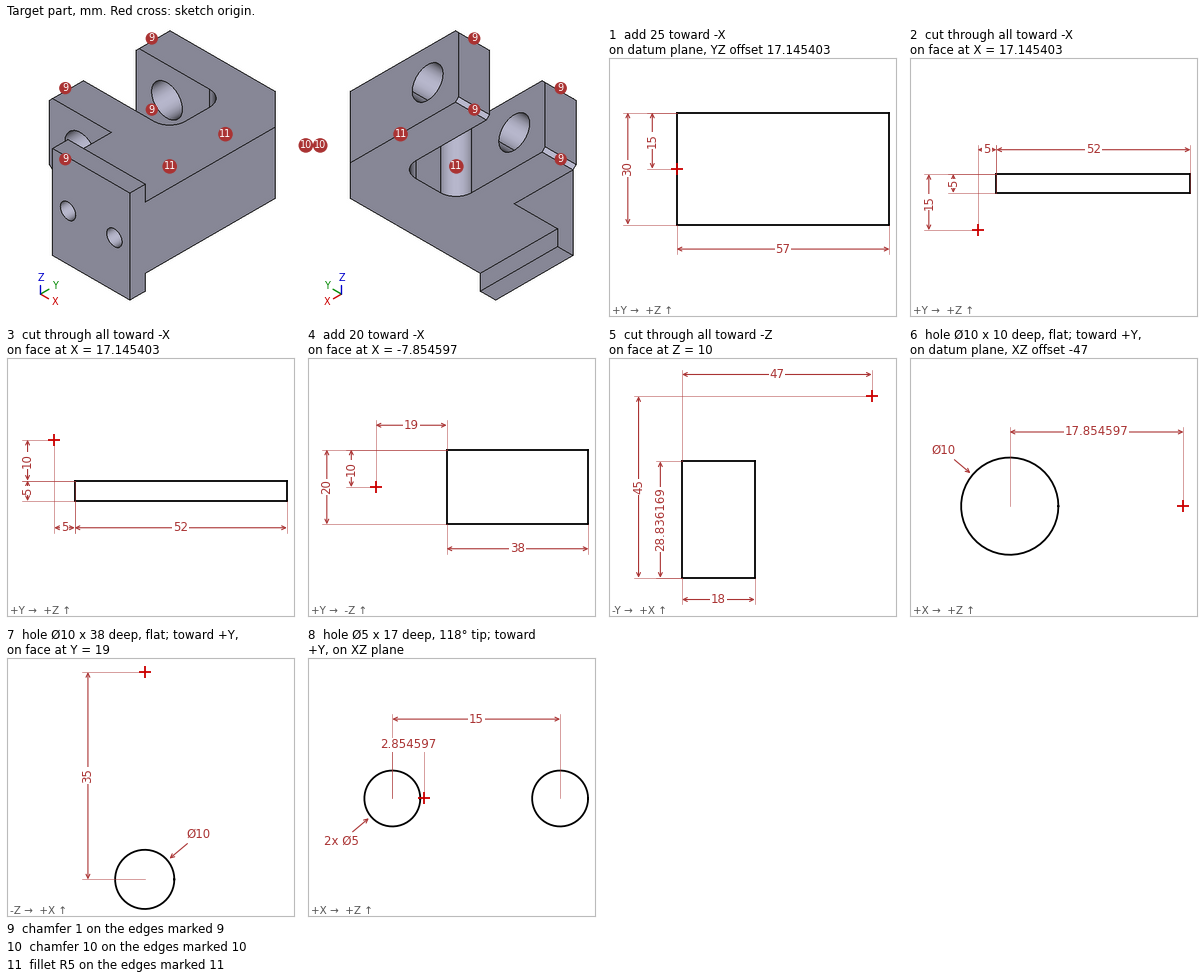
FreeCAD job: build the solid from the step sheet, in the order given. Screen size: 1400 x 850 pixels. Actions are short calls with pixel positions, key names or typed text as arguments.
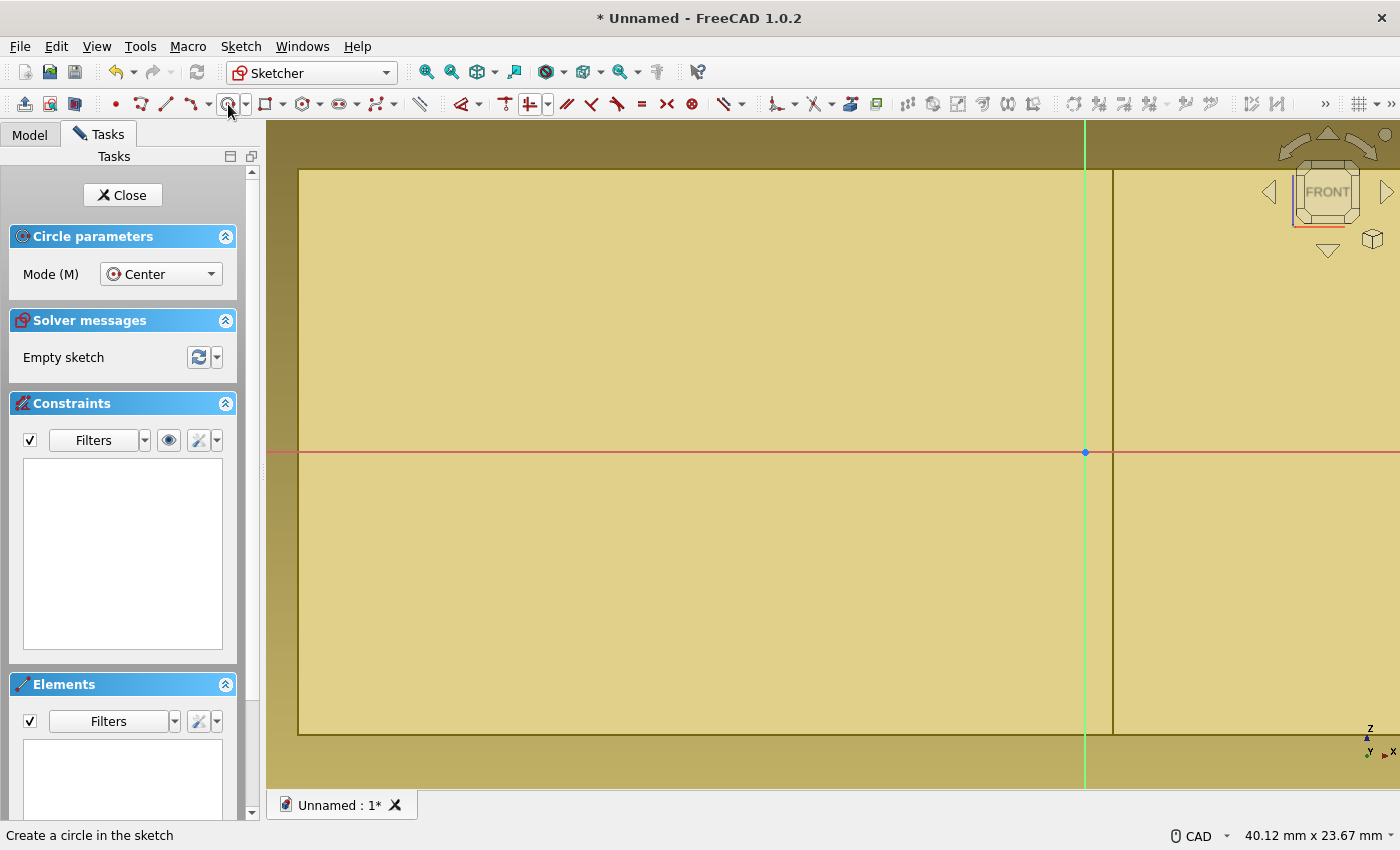
click(581, 452)
click(681, 352)
key(Escape)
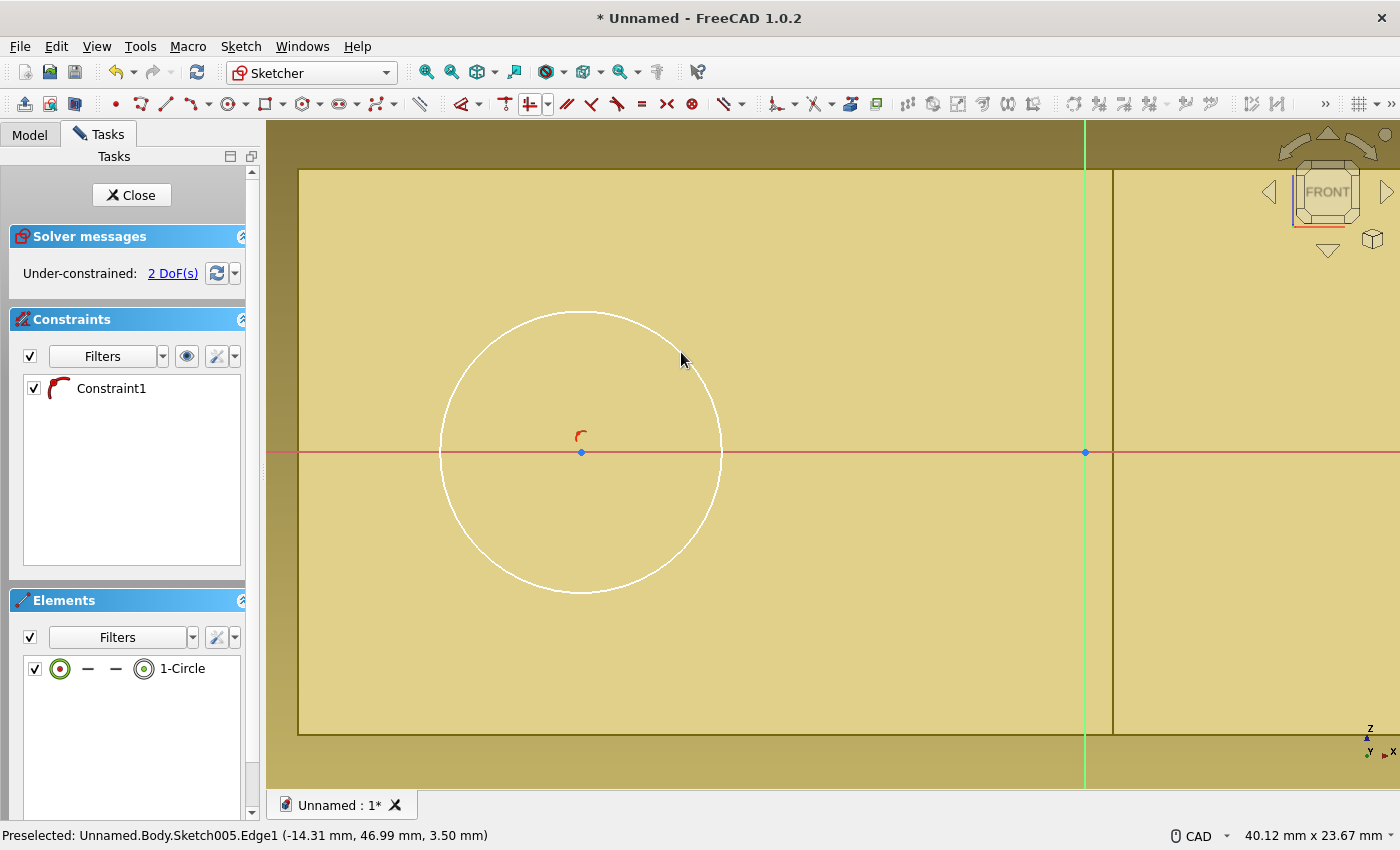
key(d)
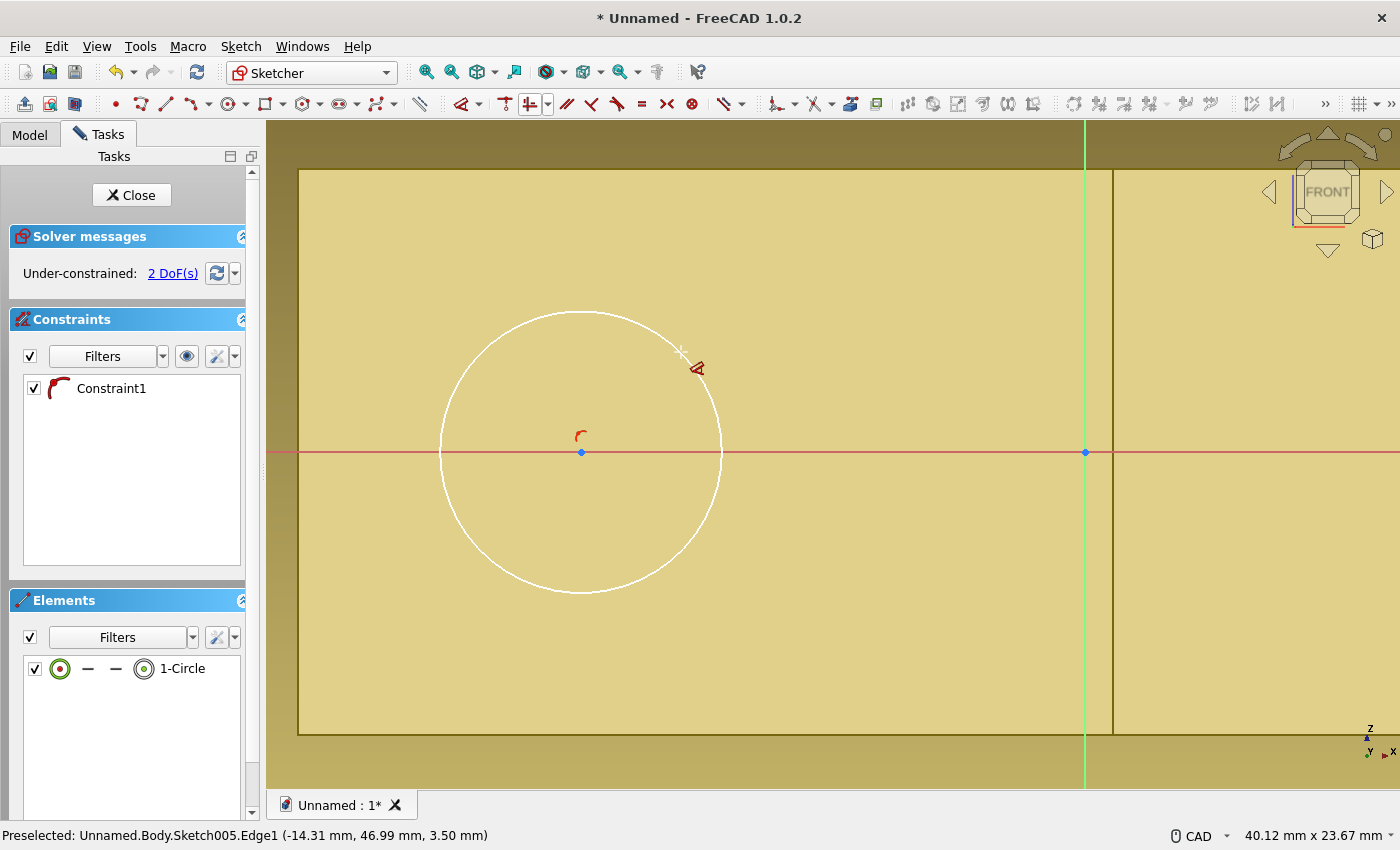
click(680, 352)
click(702, 329)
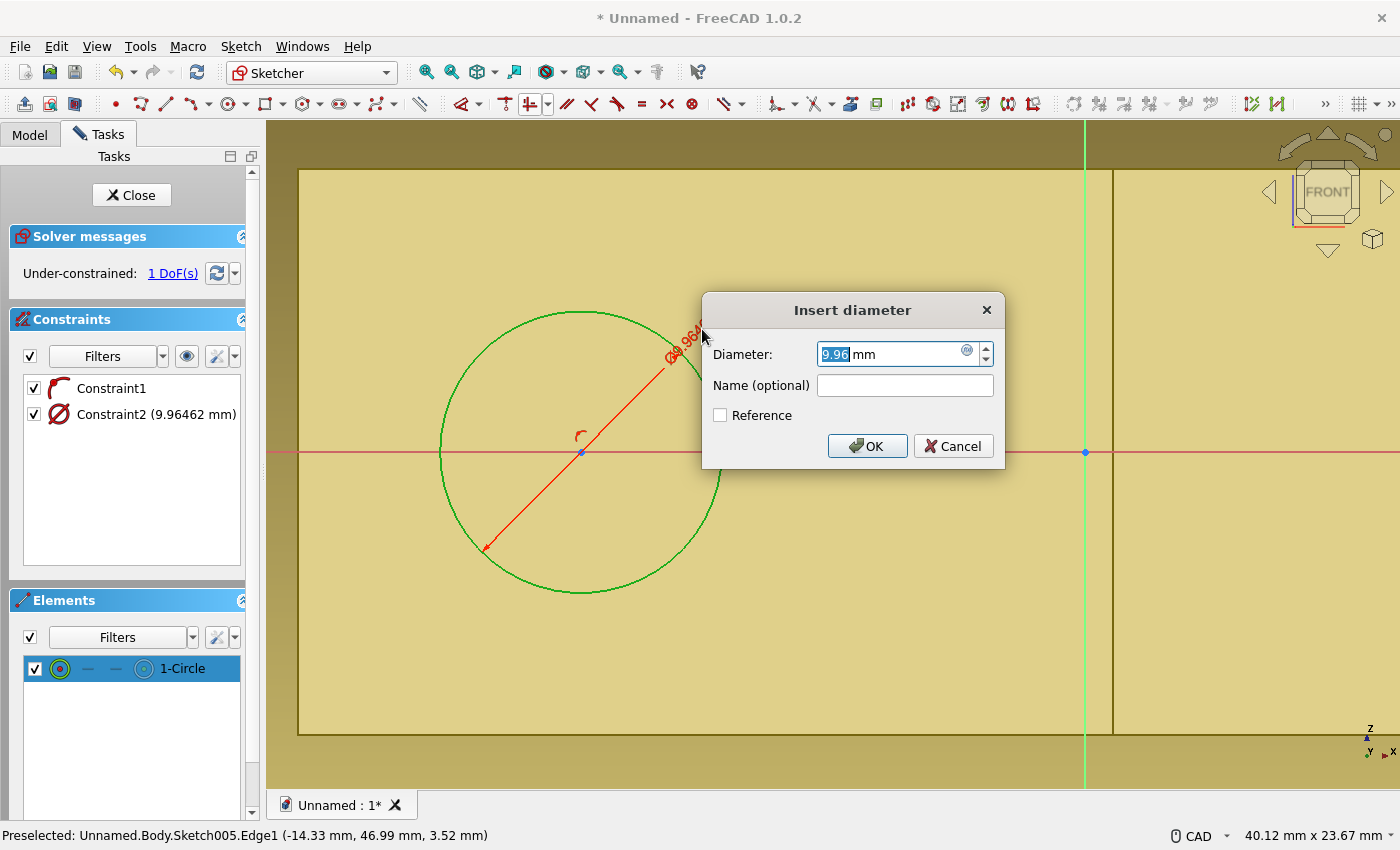
text(10)
key(Return)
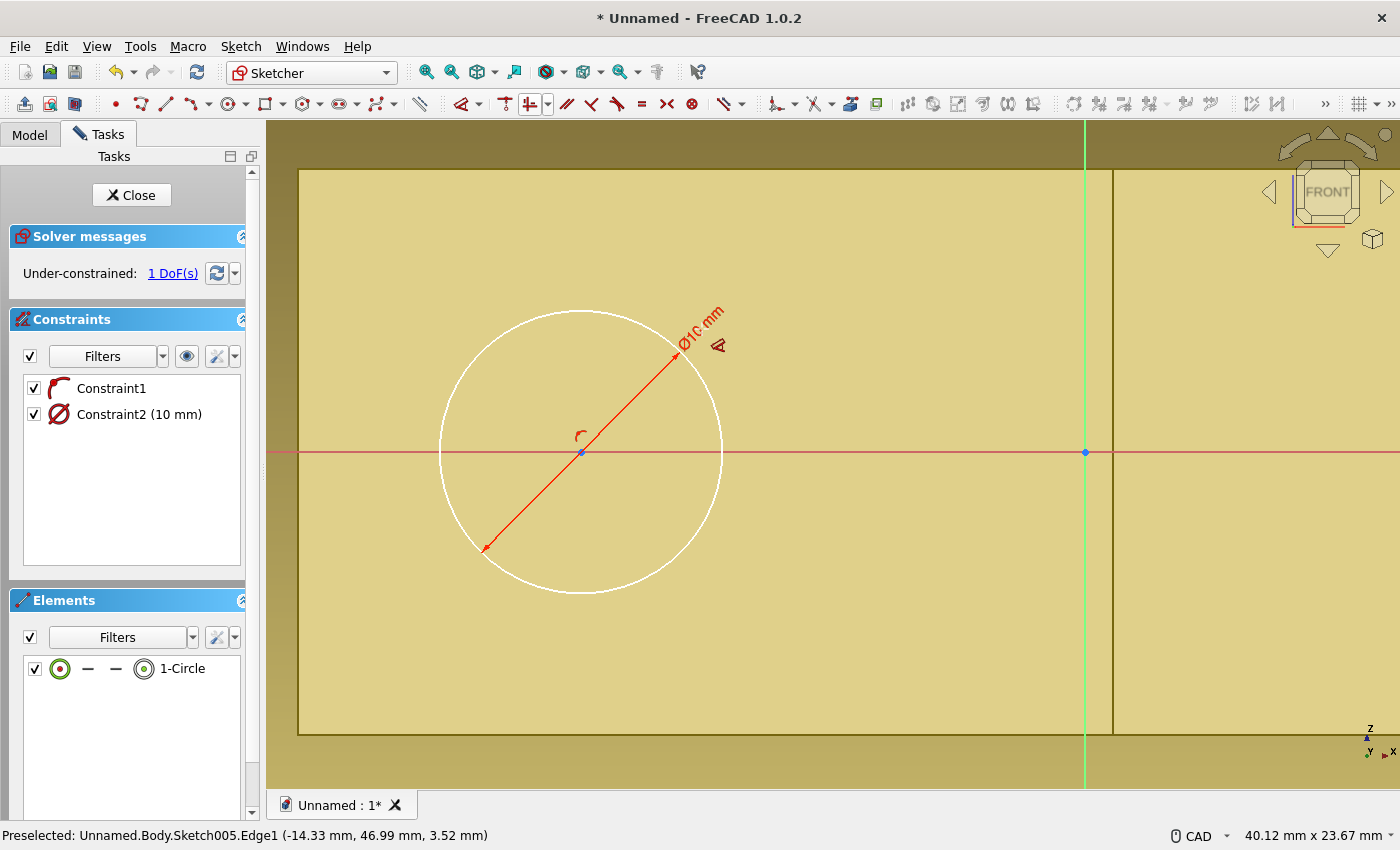
click(581, 452)
click(833, 486)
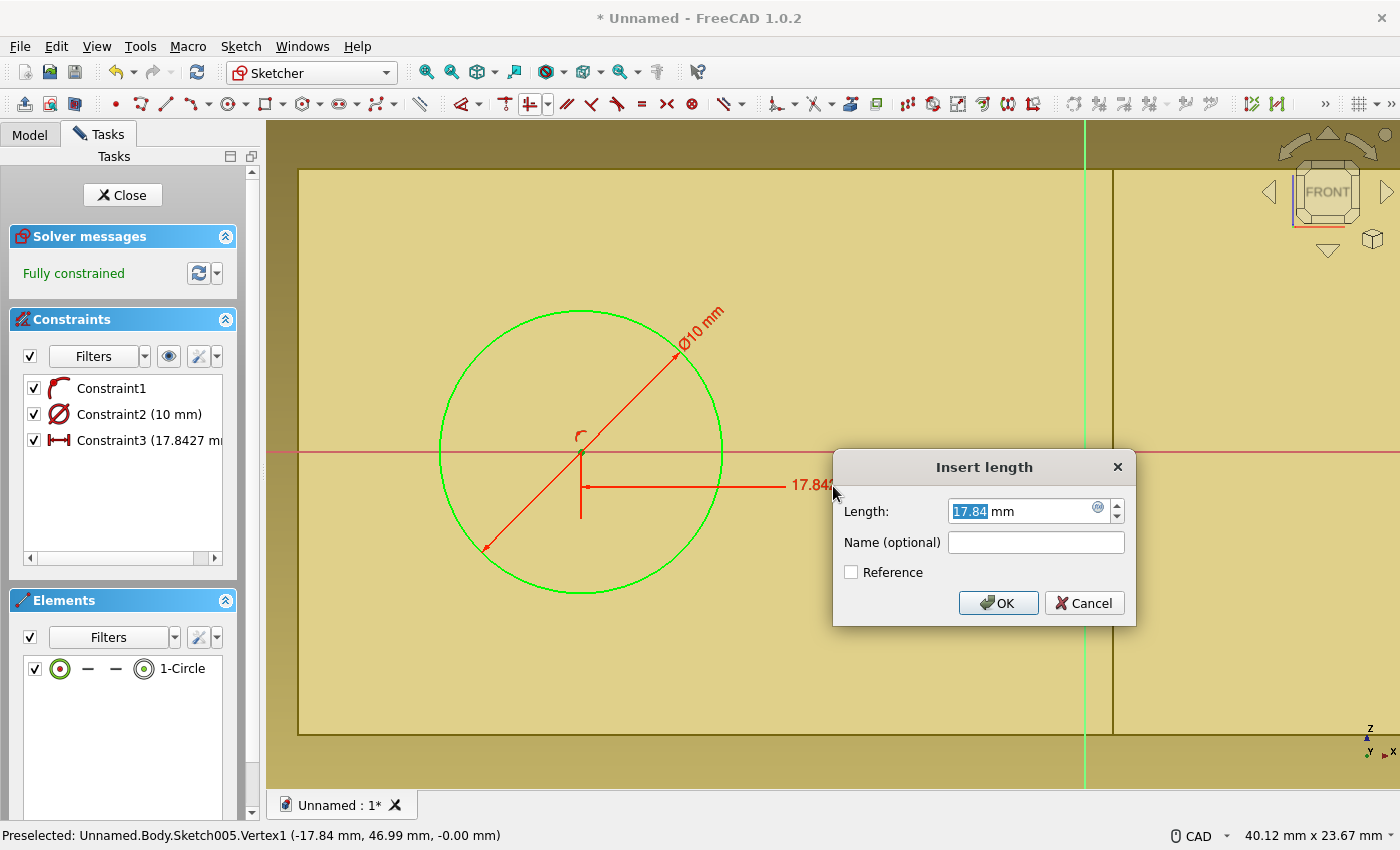
text(17.854597)
key(Return)
key(Escape)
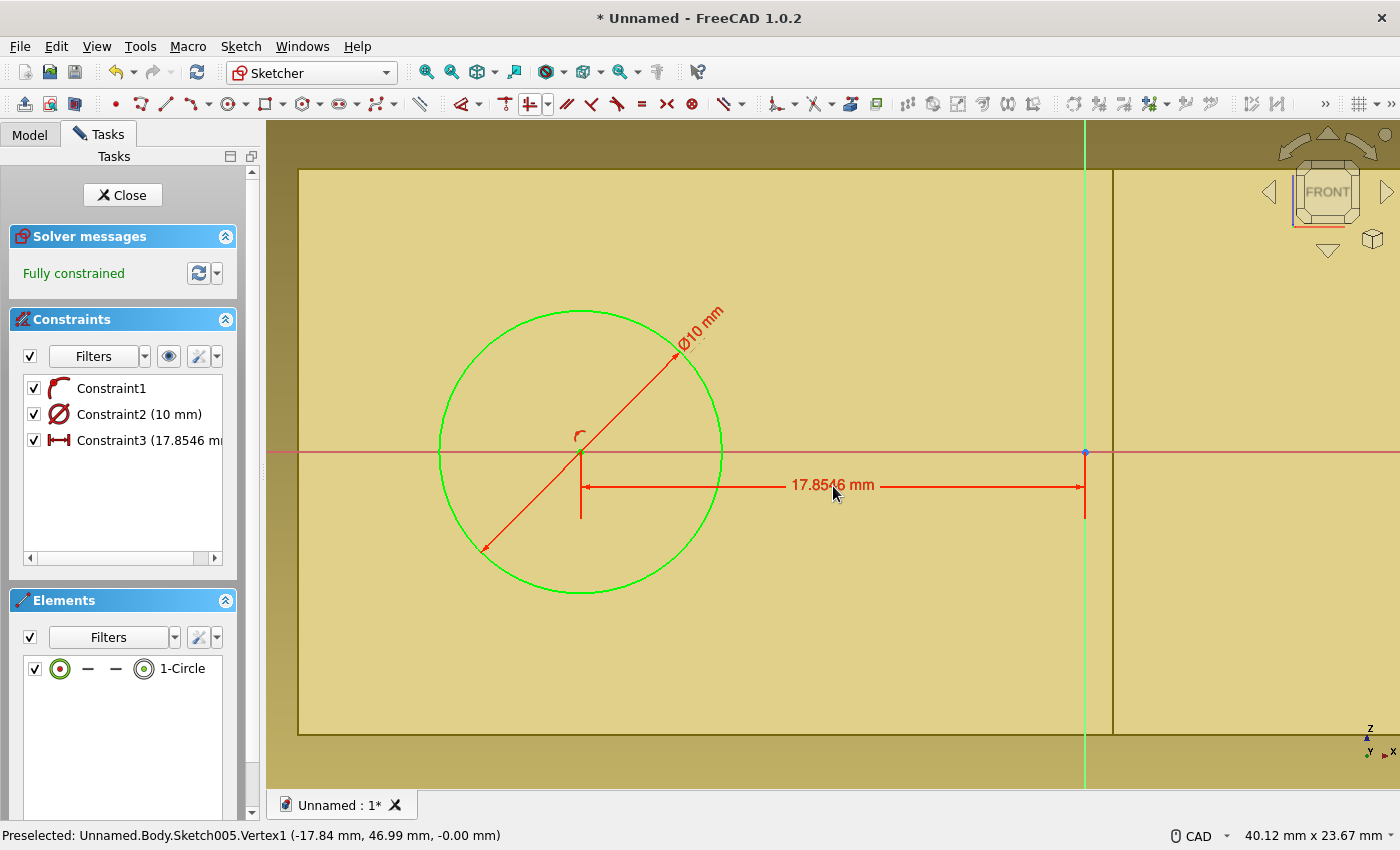
click(123, 195)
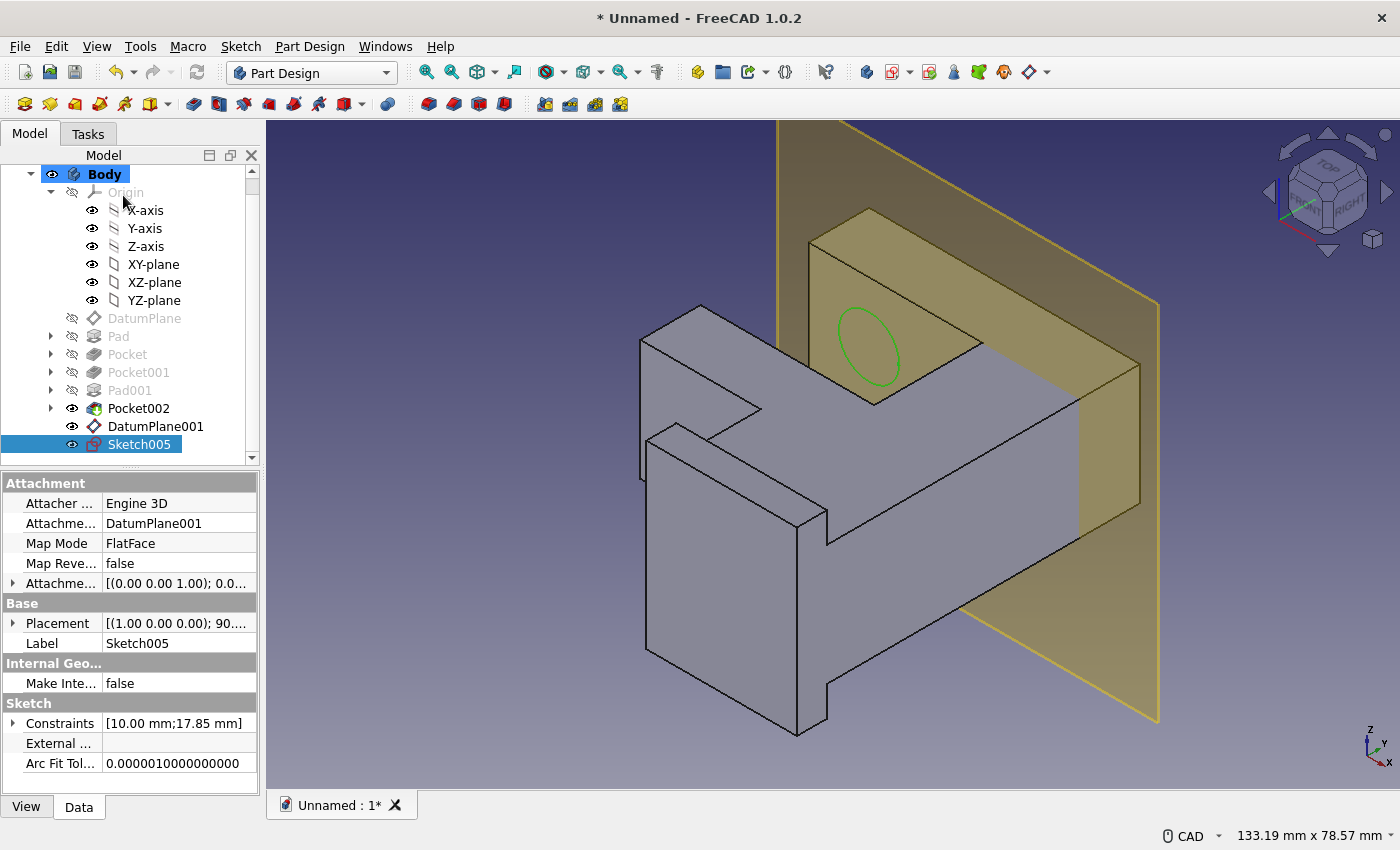
click(219, 104)